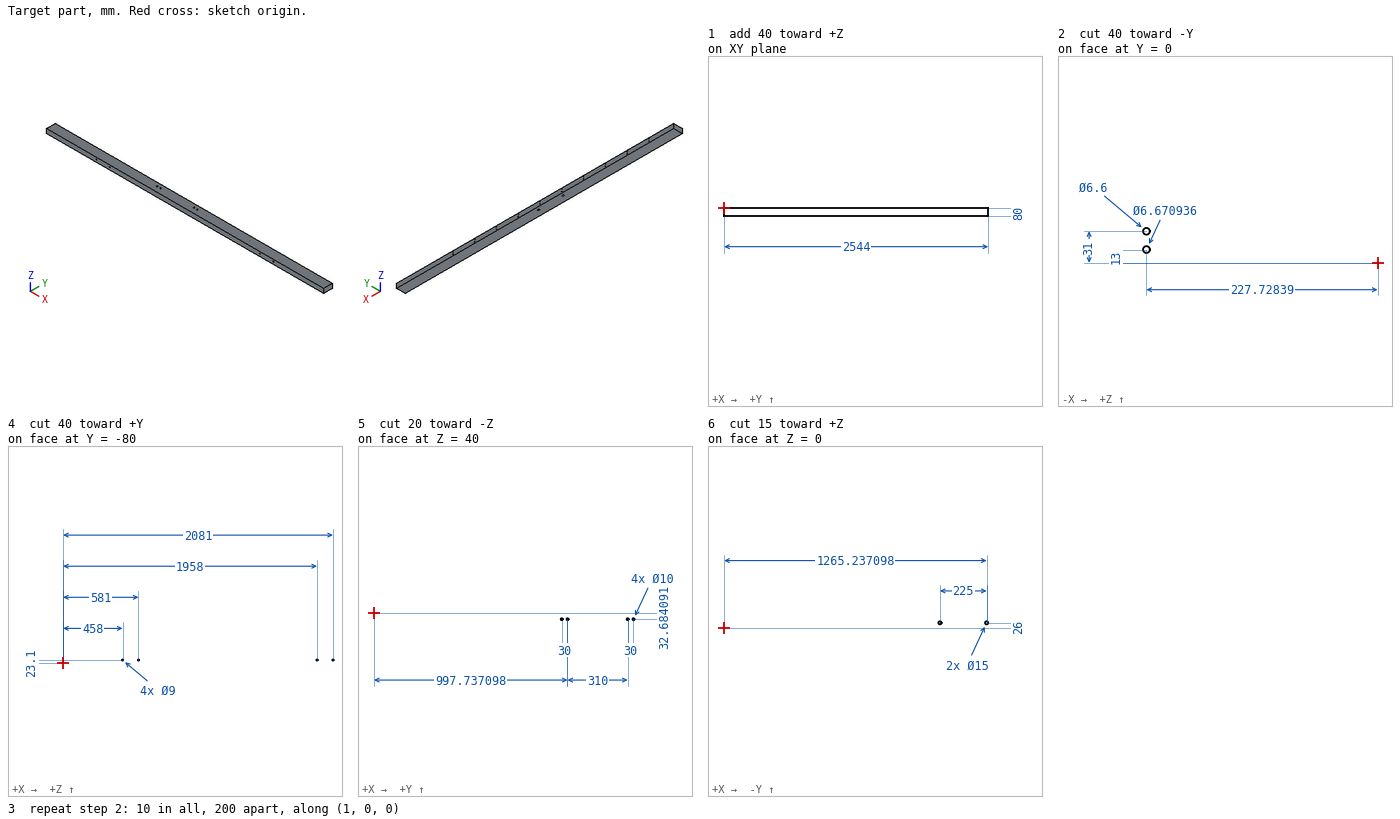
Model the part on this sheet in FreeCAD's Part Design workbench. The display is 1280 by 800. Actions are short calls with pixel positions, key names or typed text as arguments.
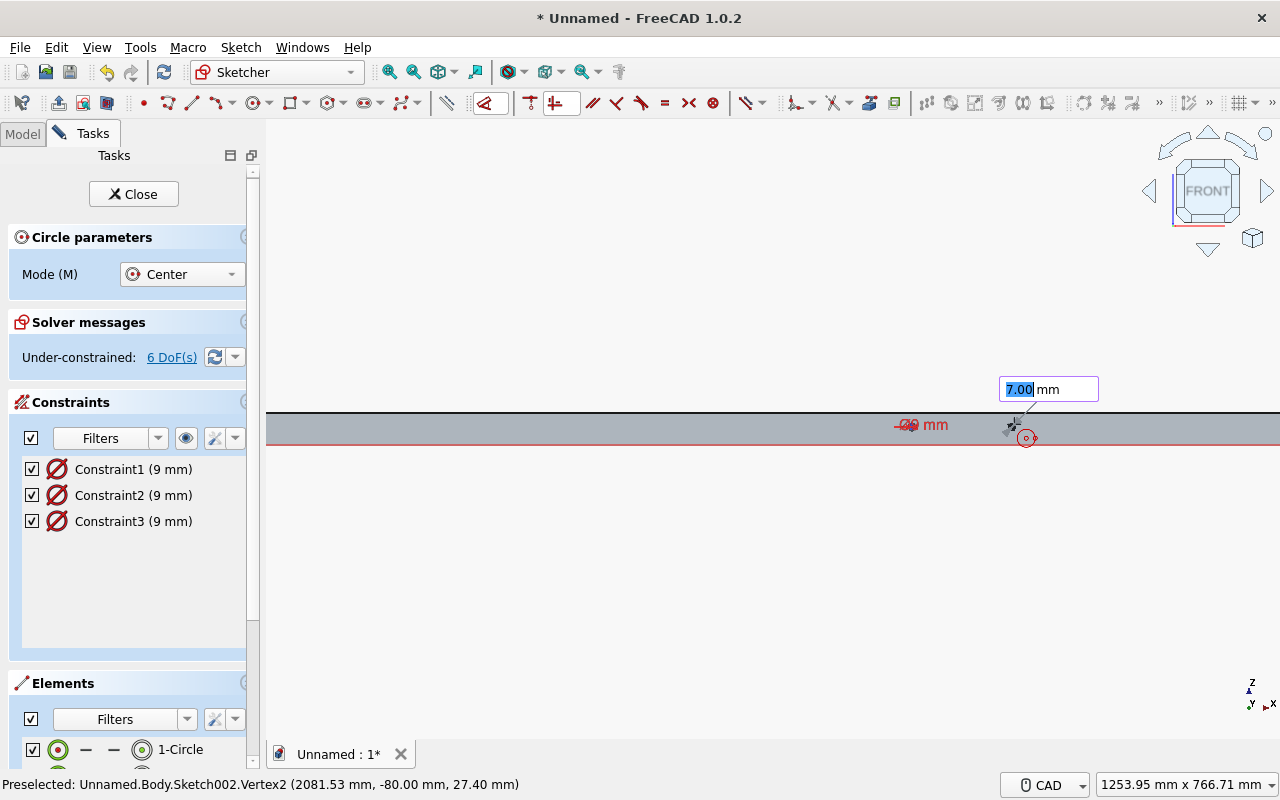
text(9)
key(Return)
key(Escape)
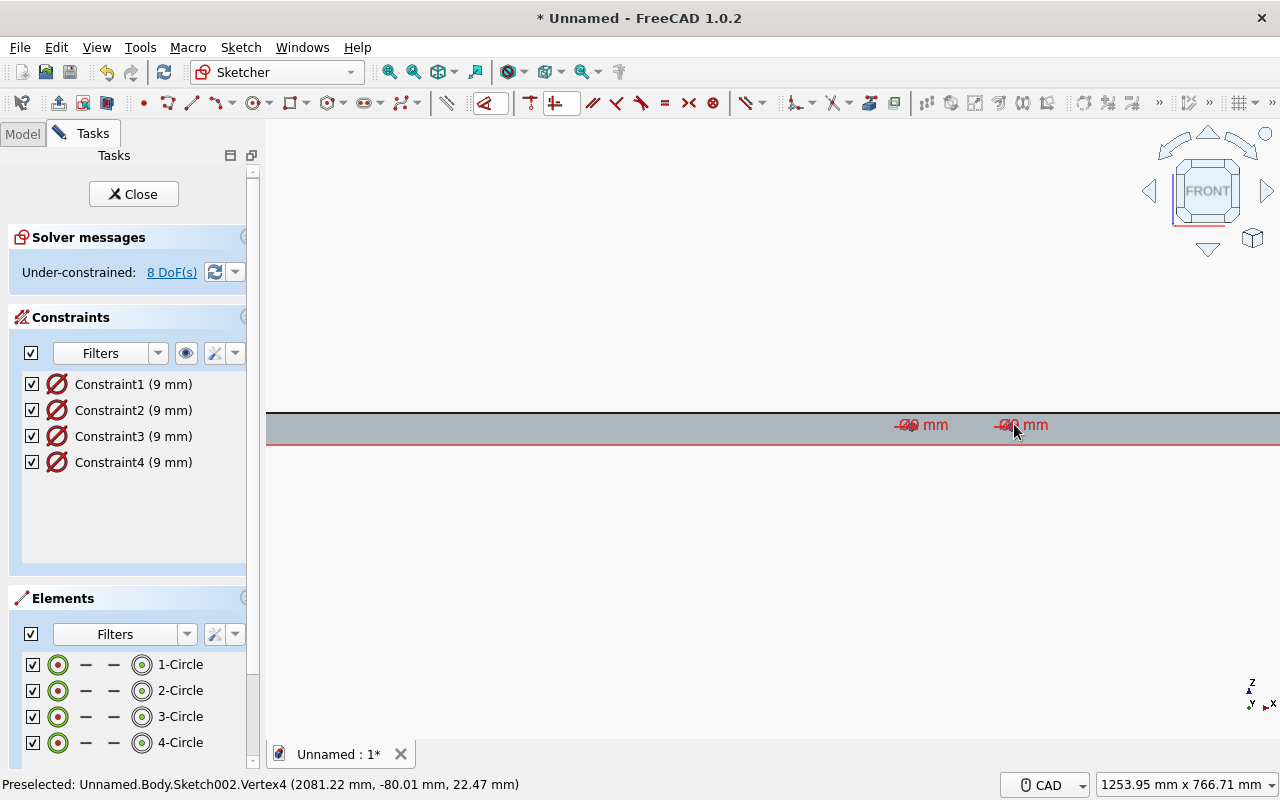
scroll(1014, 426, down, 5)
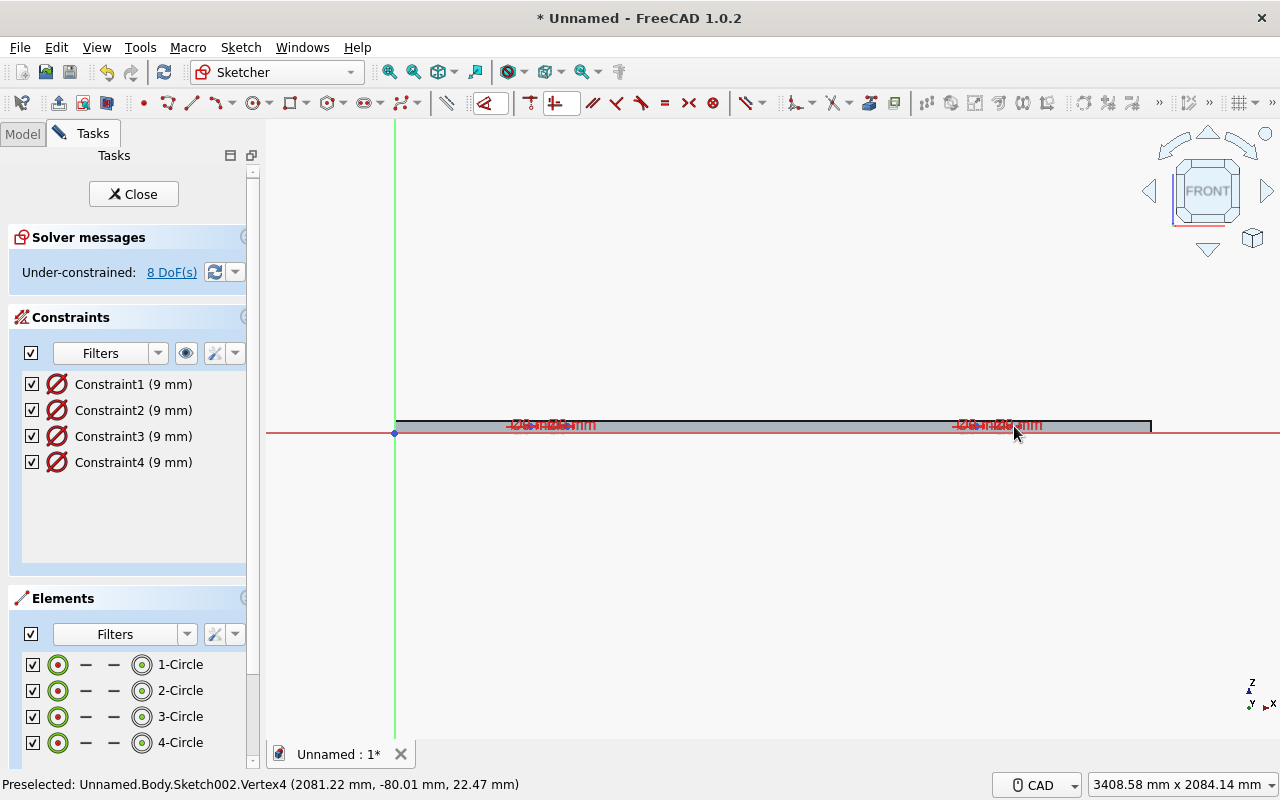
click(531, 427)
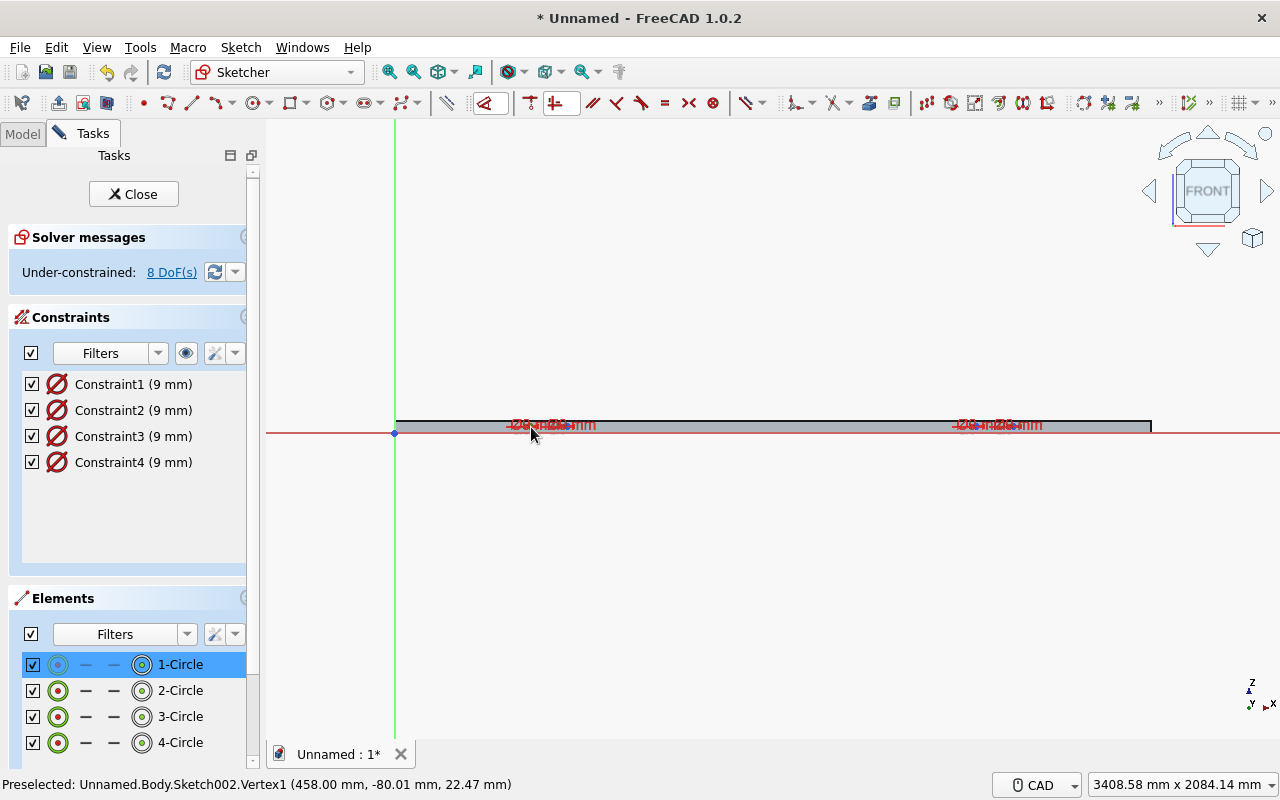
click(567, 427)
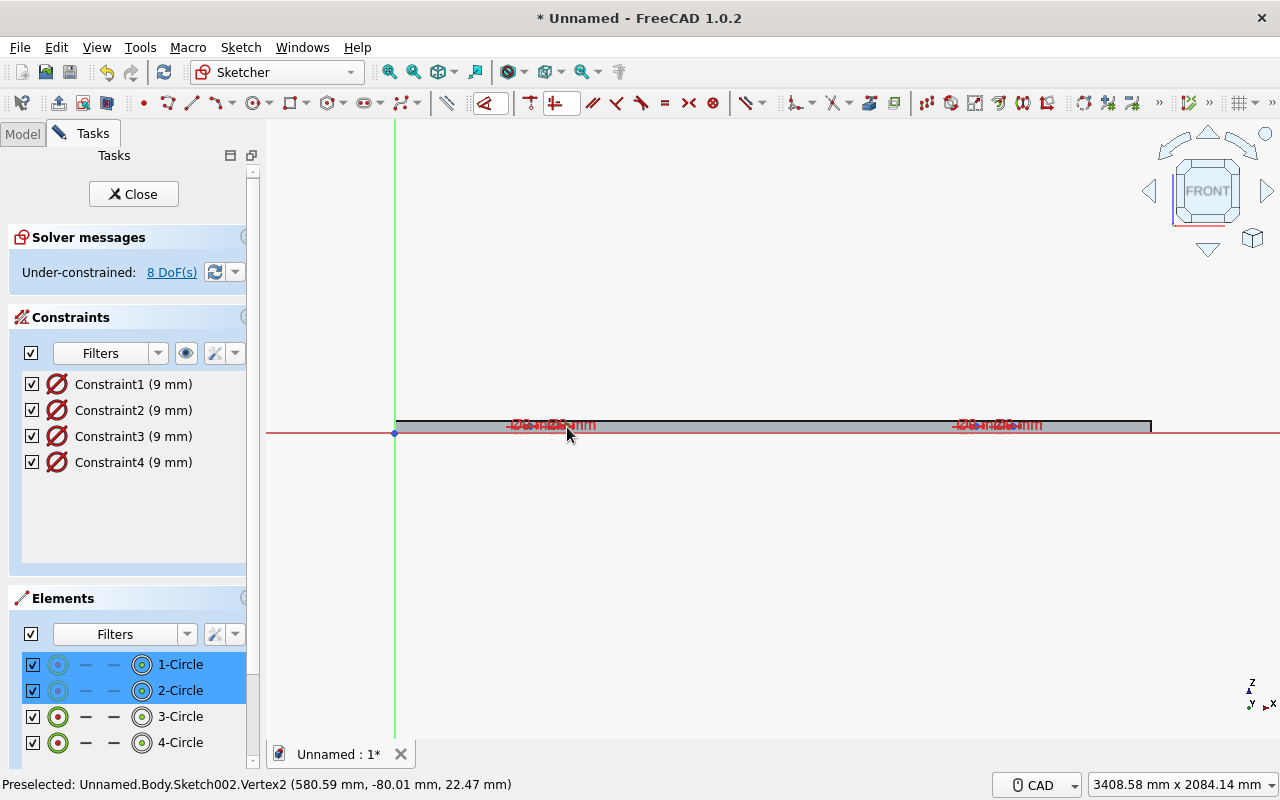
key(h)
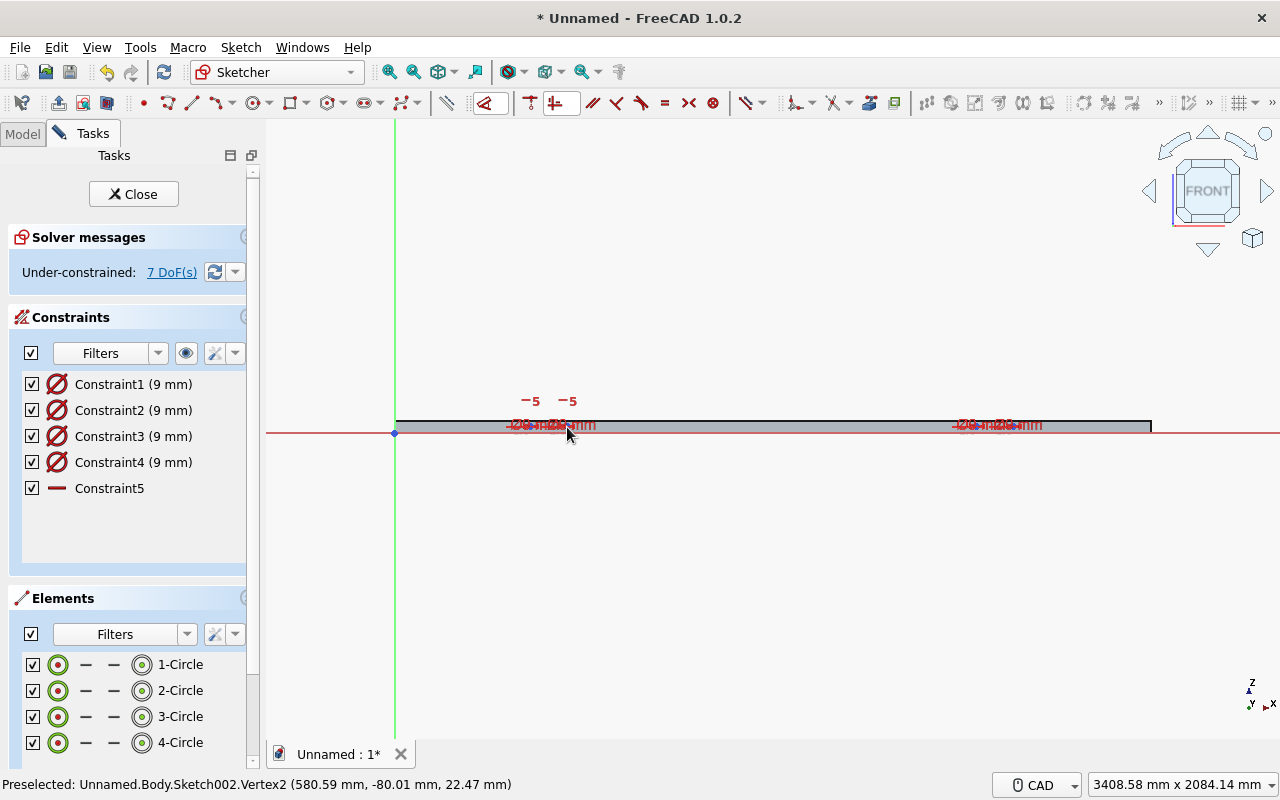
click(567, 427)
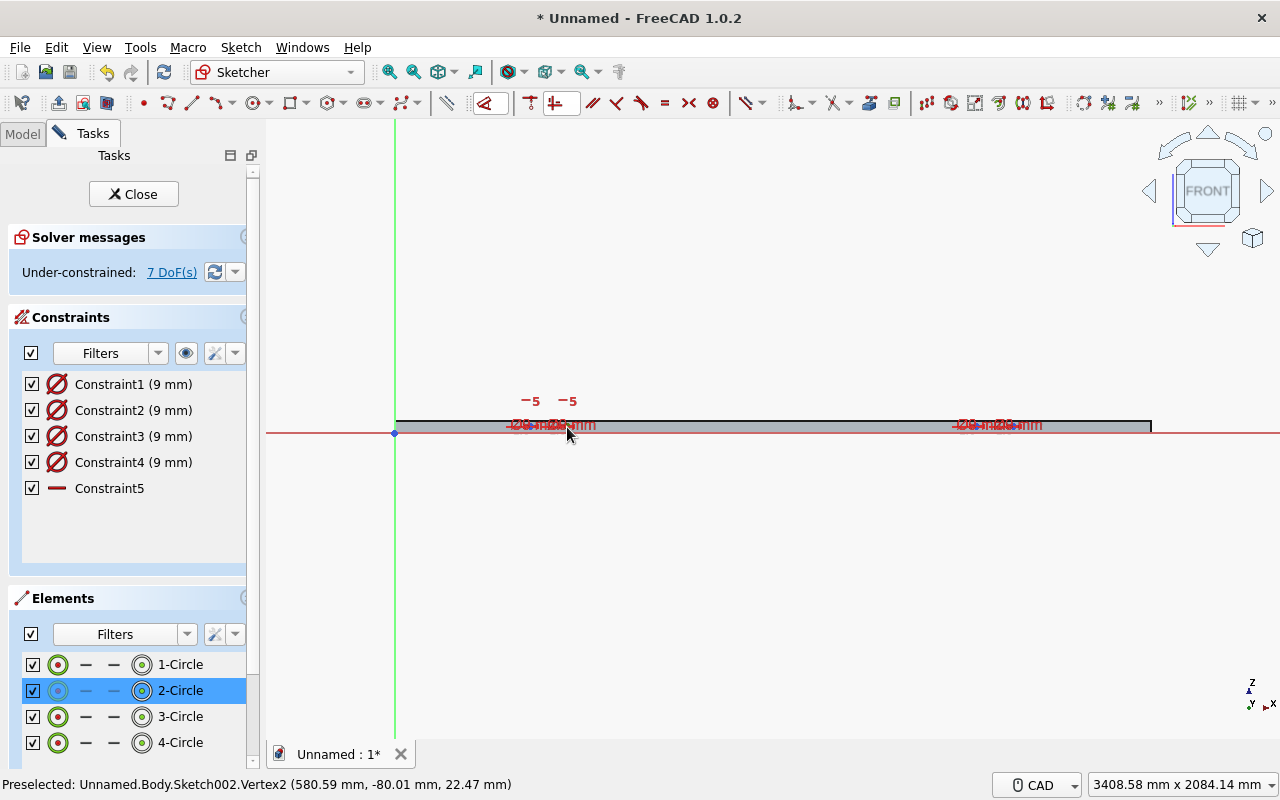
click(977, 427)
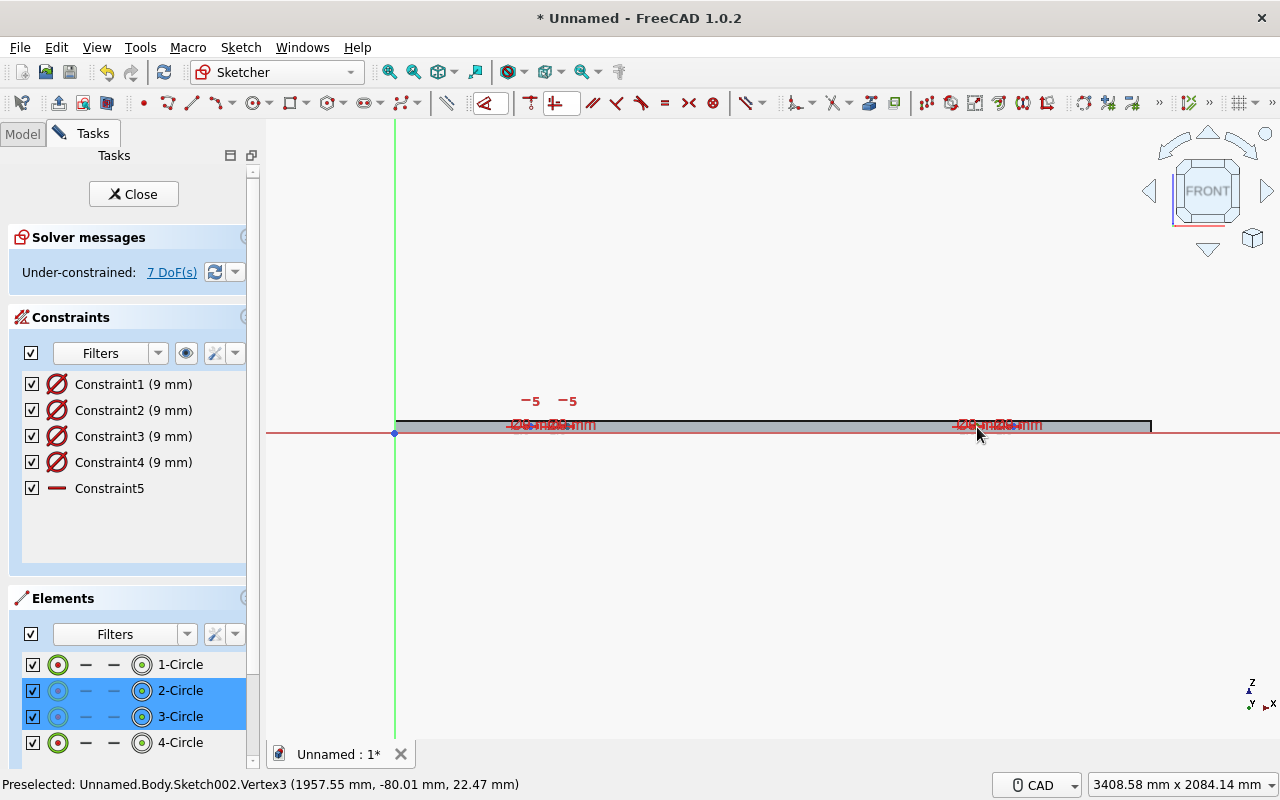
key(h)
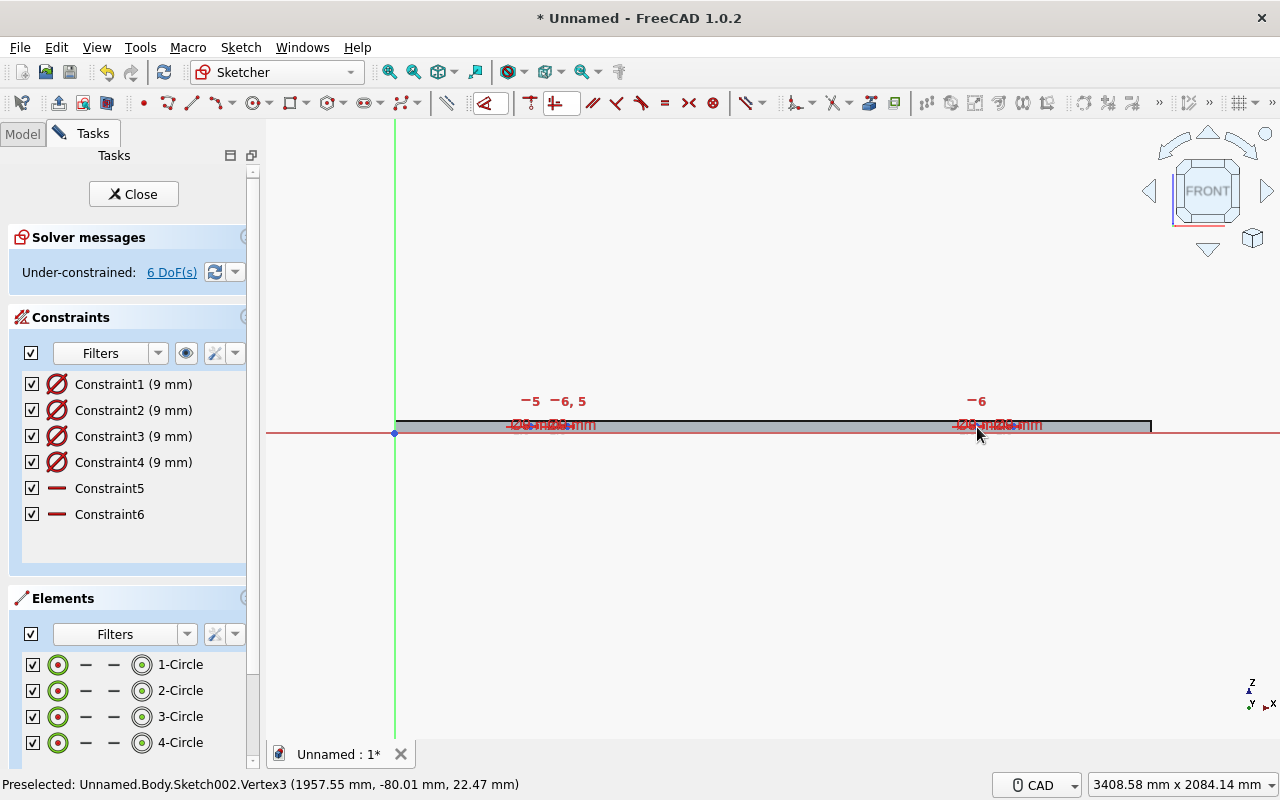
click(977, 427)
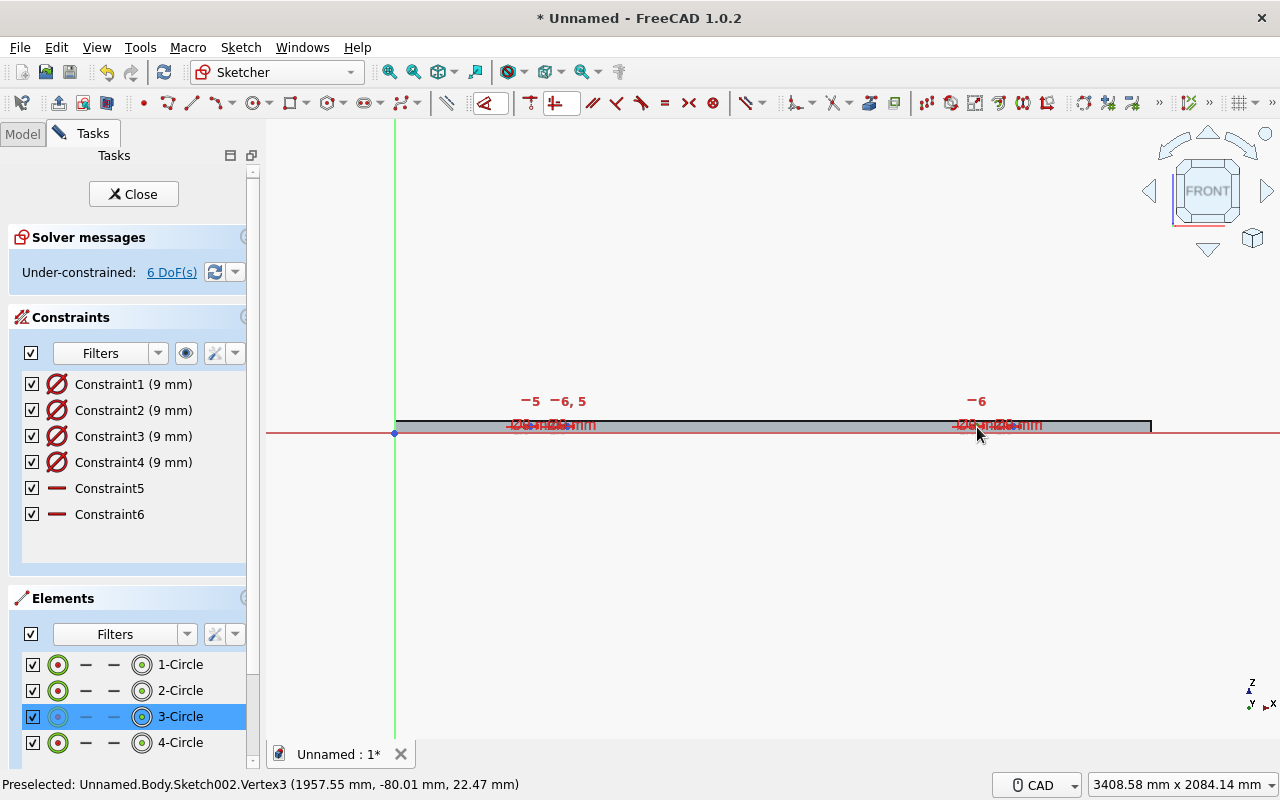
click(1014, 427)